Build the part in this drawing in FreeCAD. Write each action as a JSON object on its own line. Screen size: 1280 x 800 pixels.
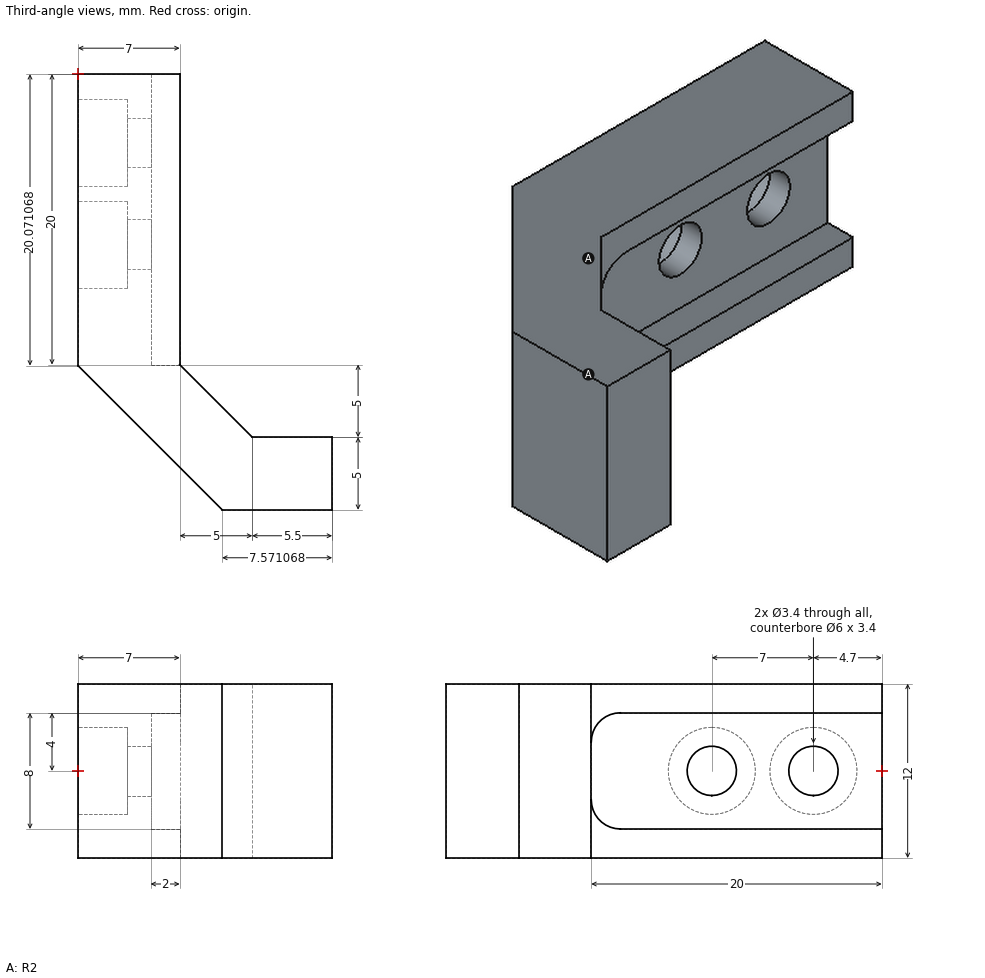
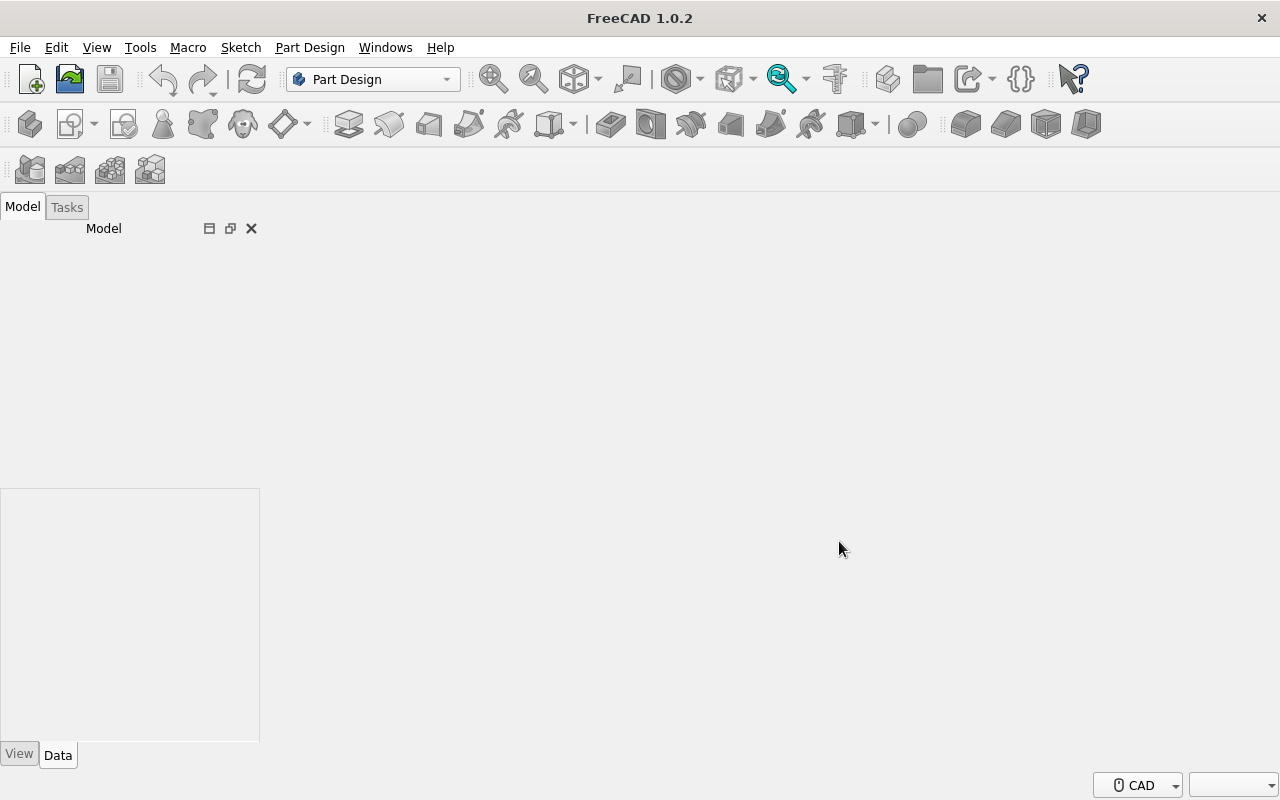
{"action": "left_click", "coordinate": [30, 80]}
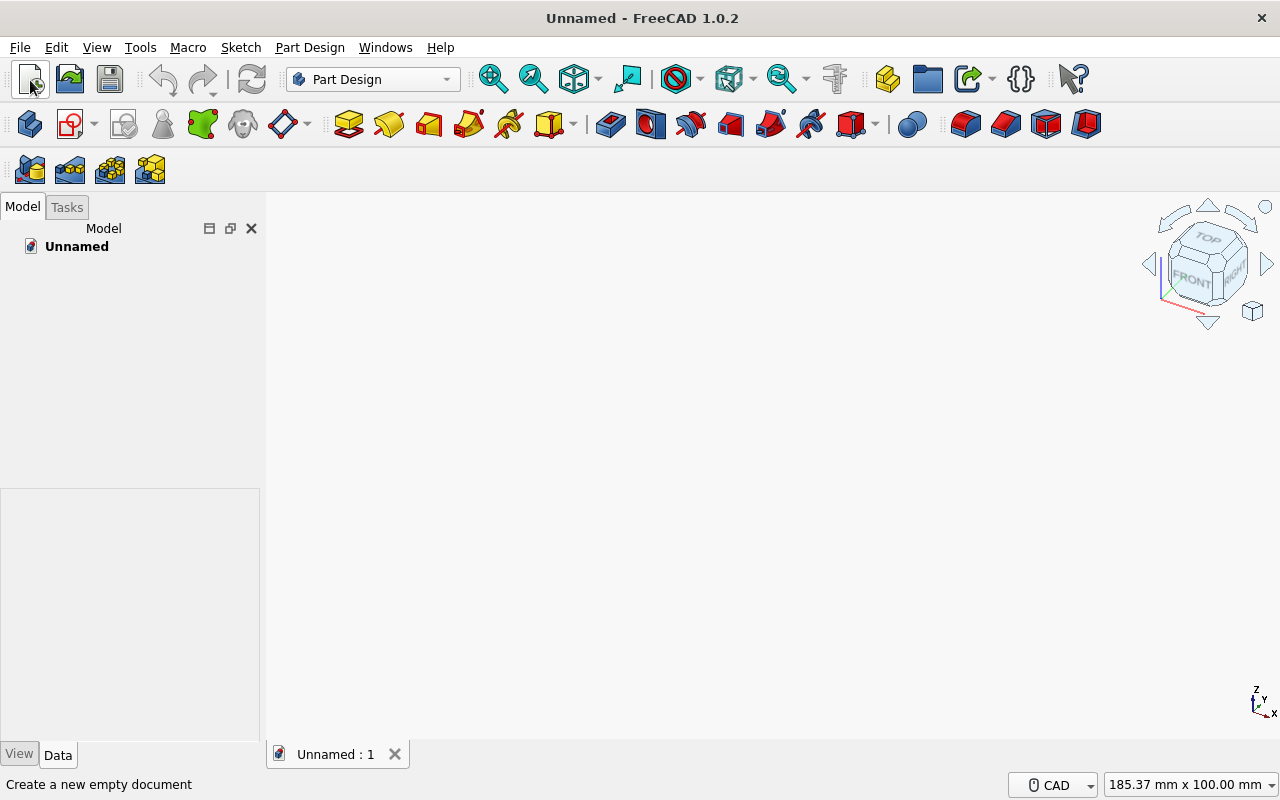
{"action": "left_click", "coordinate": [70, 124]}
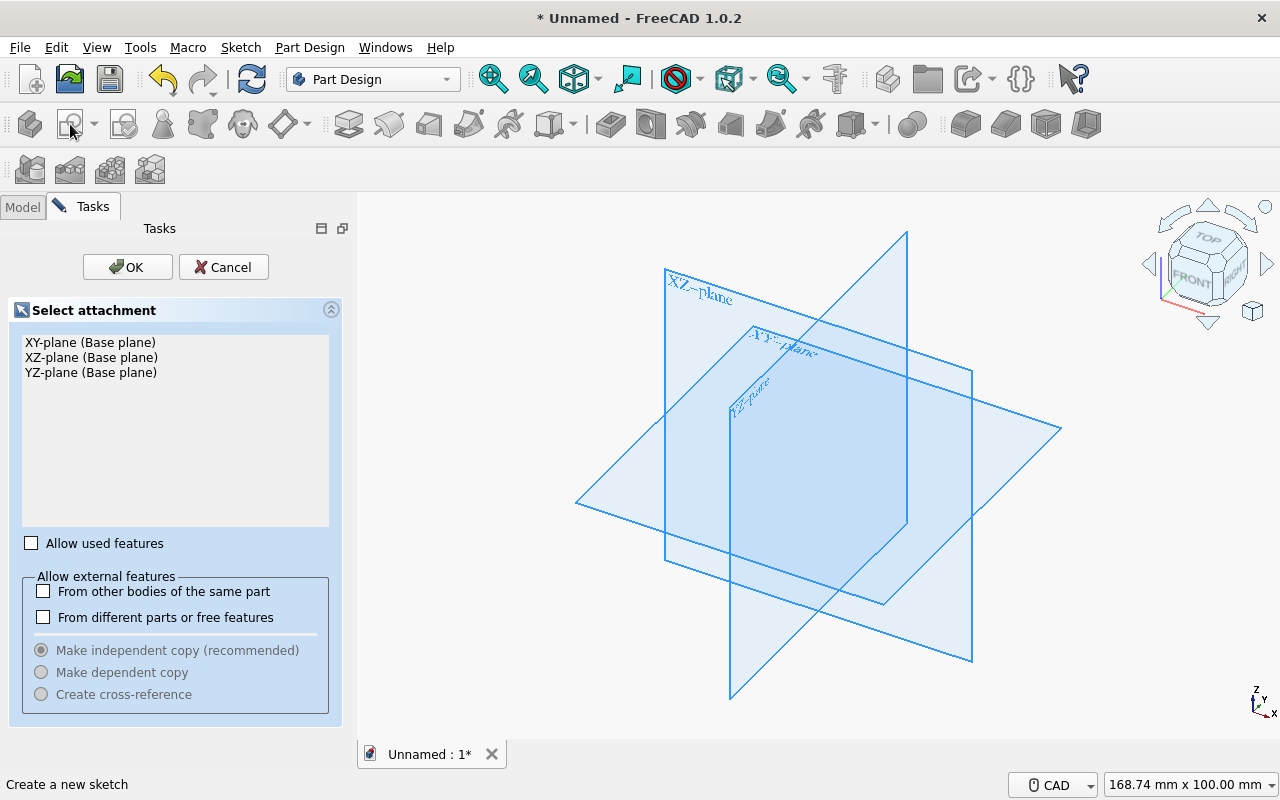
{"action": "left_click", "coordinate": [82, 342]}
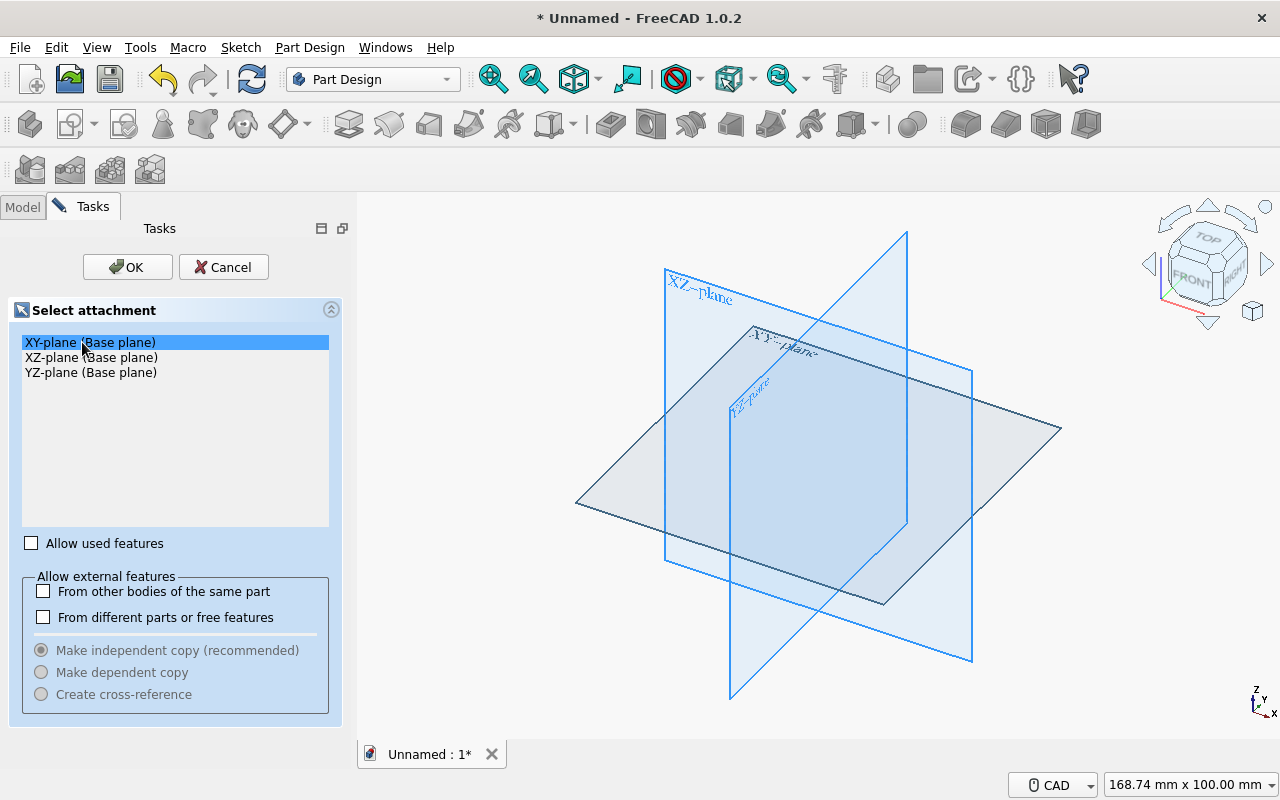
{"action": "left_click", "coordinate": [128, 267]}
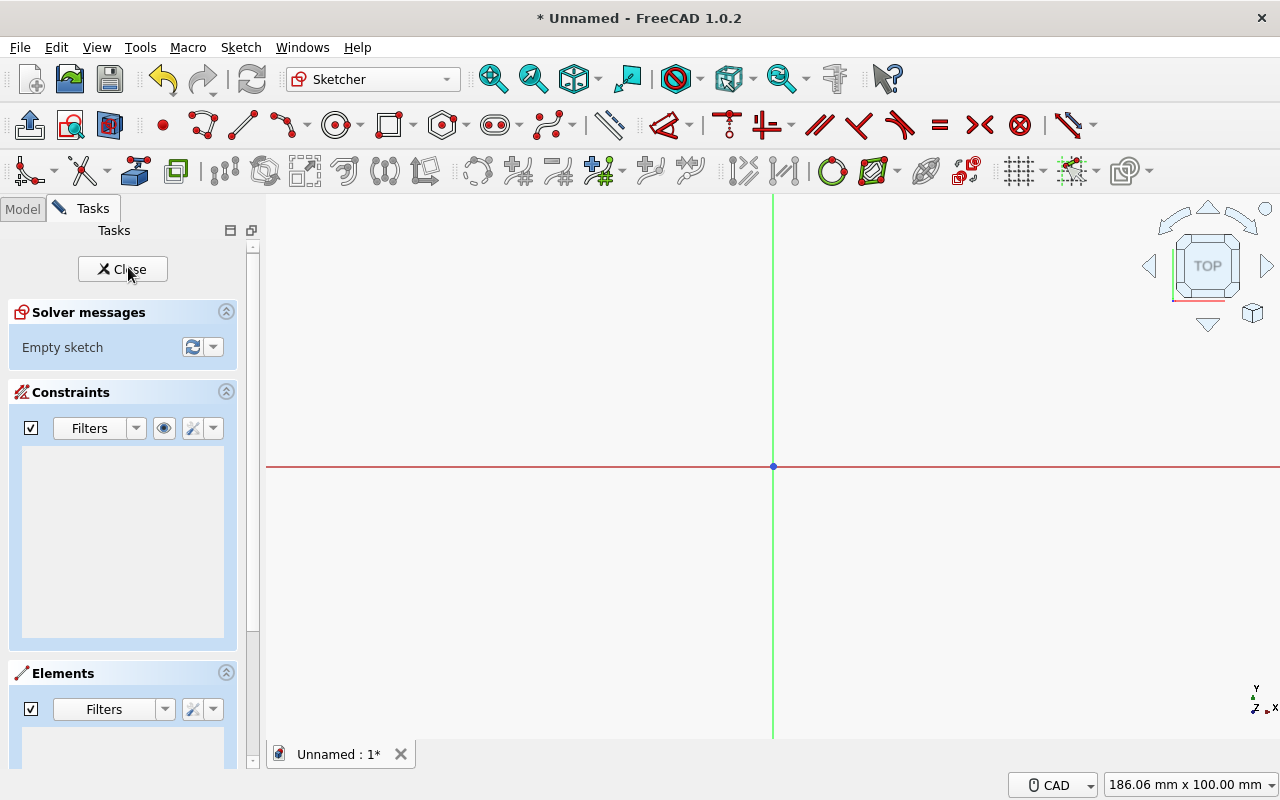
{"action": "scroll", "coordinate": [915, 615], "scroll_direction": "up", "scroll_amount": 4}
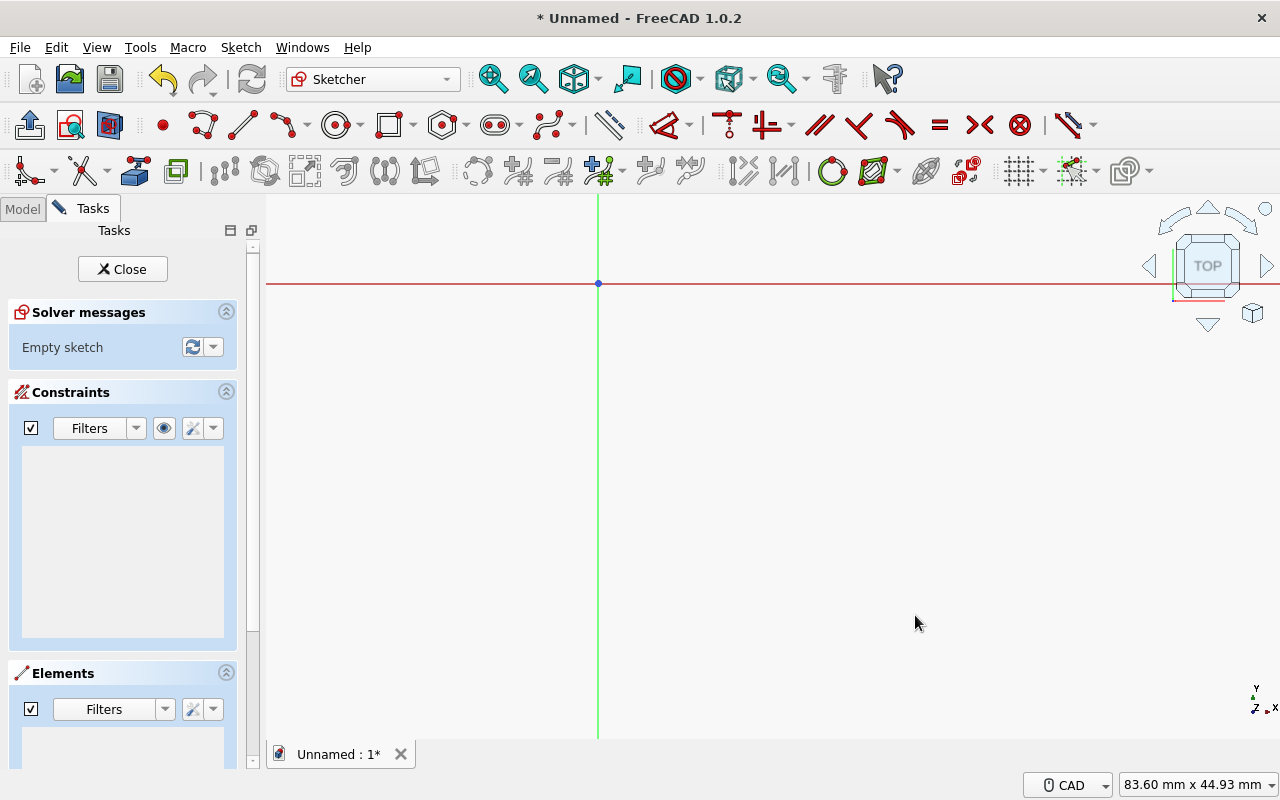
{"action": "left_click", "coordinate": [204, 126]}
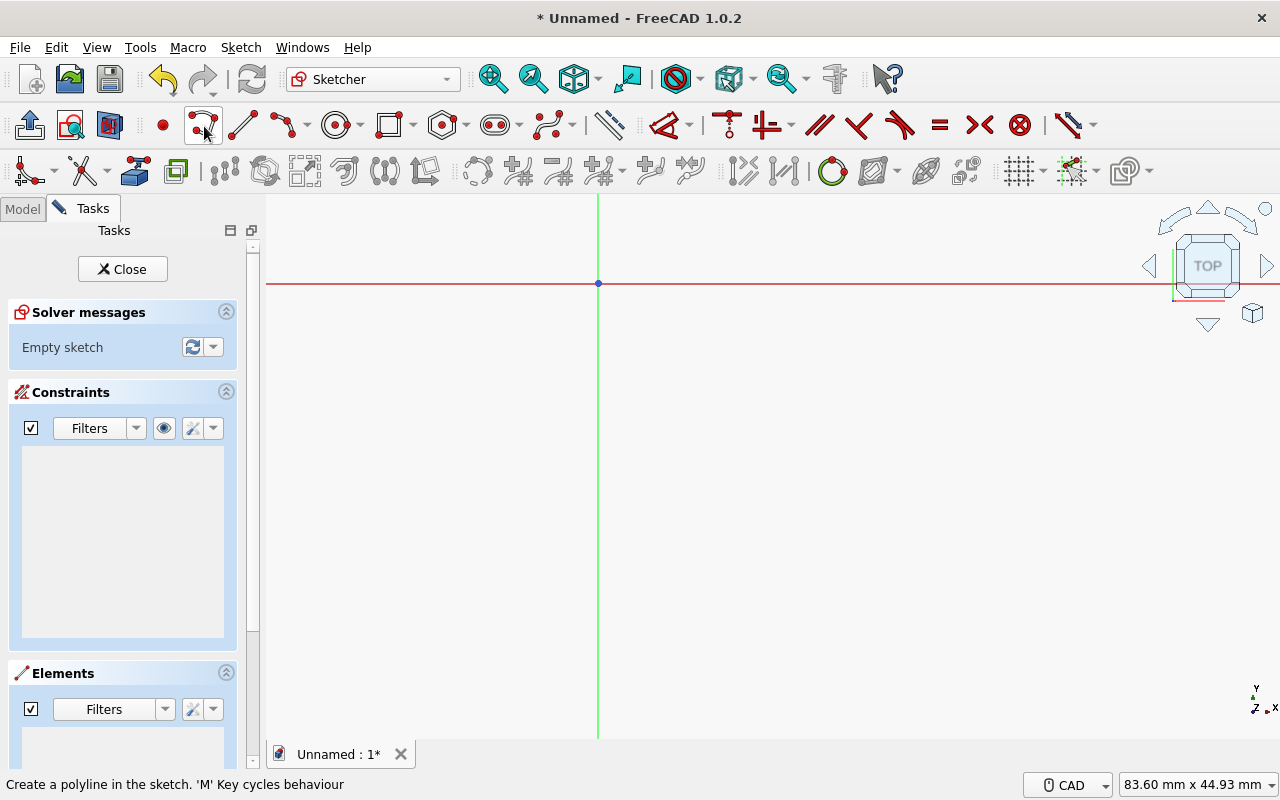
{"action": "left_click", "coordinate": [598, 284]}
{"action": "left_click", "coordinate": [607, 527]}
{"action": "left_click", "coordinate": [719, 647]}
{"action": "left_click", "coordinate": [810, 647]}
{"action": "left_click", "coordinate": [810, 587]}
{"action": "left_click", "coordinate": [744, 587]}
{"action": "left_click", "coordinate": [683, 526]}
{"action": "left_click", "coordinate": [683, 293]}
{"action": "left_click", "coordinate": [598, 284]}
{"action": "key", "text": "Escape"}
{"action": "key", "text": "Escape"}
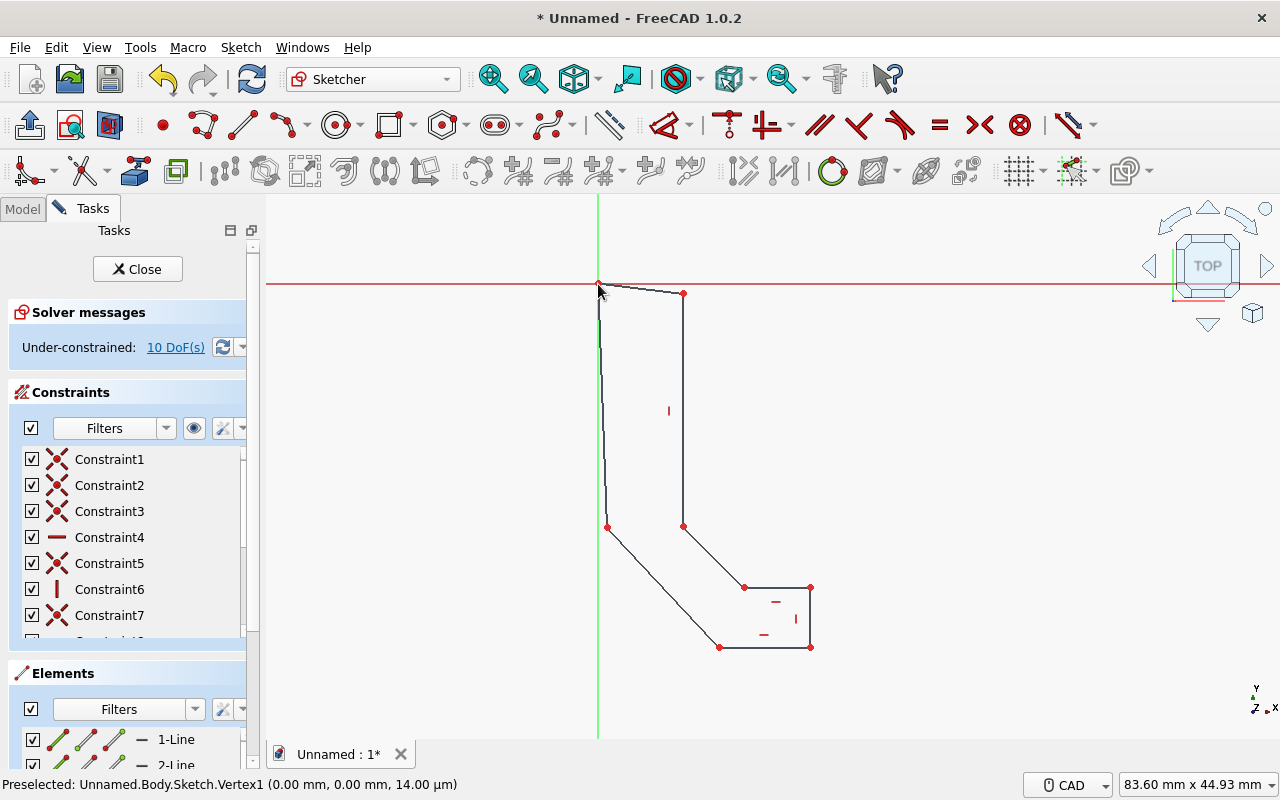
{"action": "left_click", "coordinate": [601, 357]}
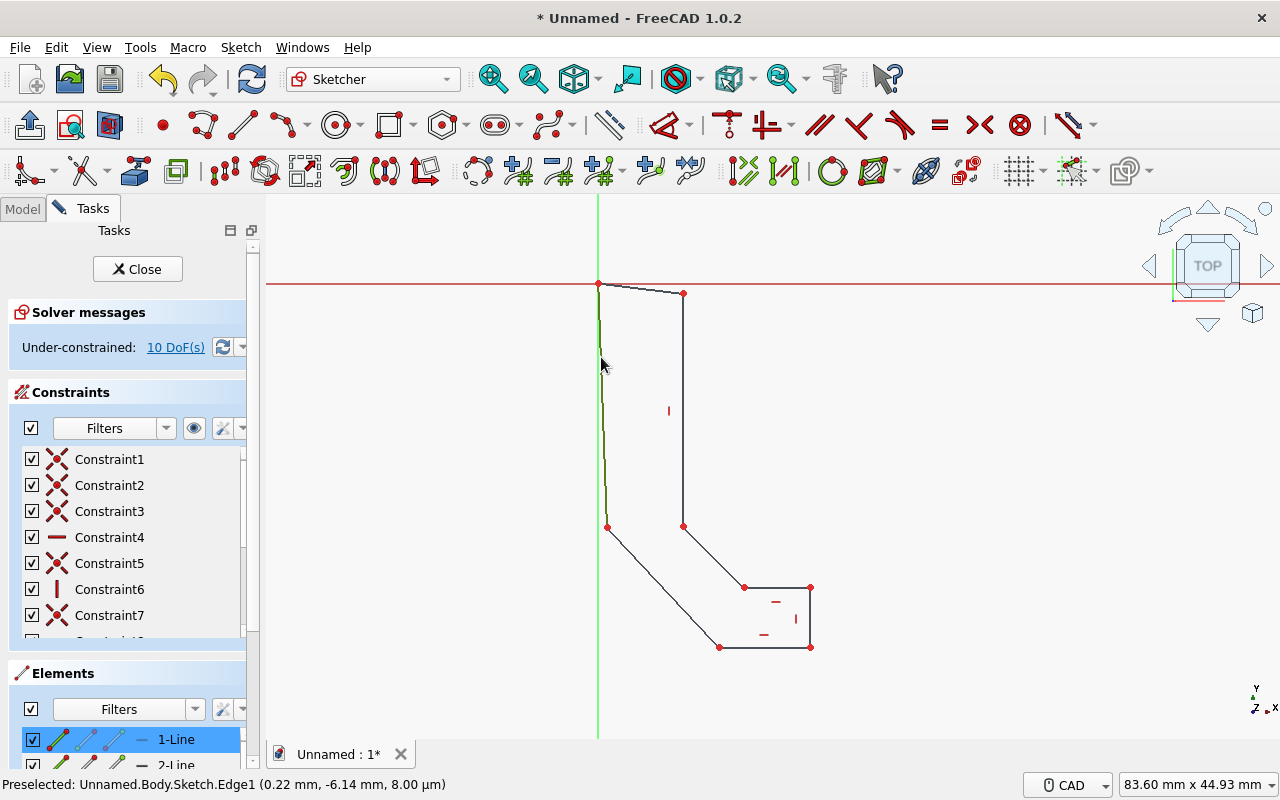
{"action": "key", "text": "v"}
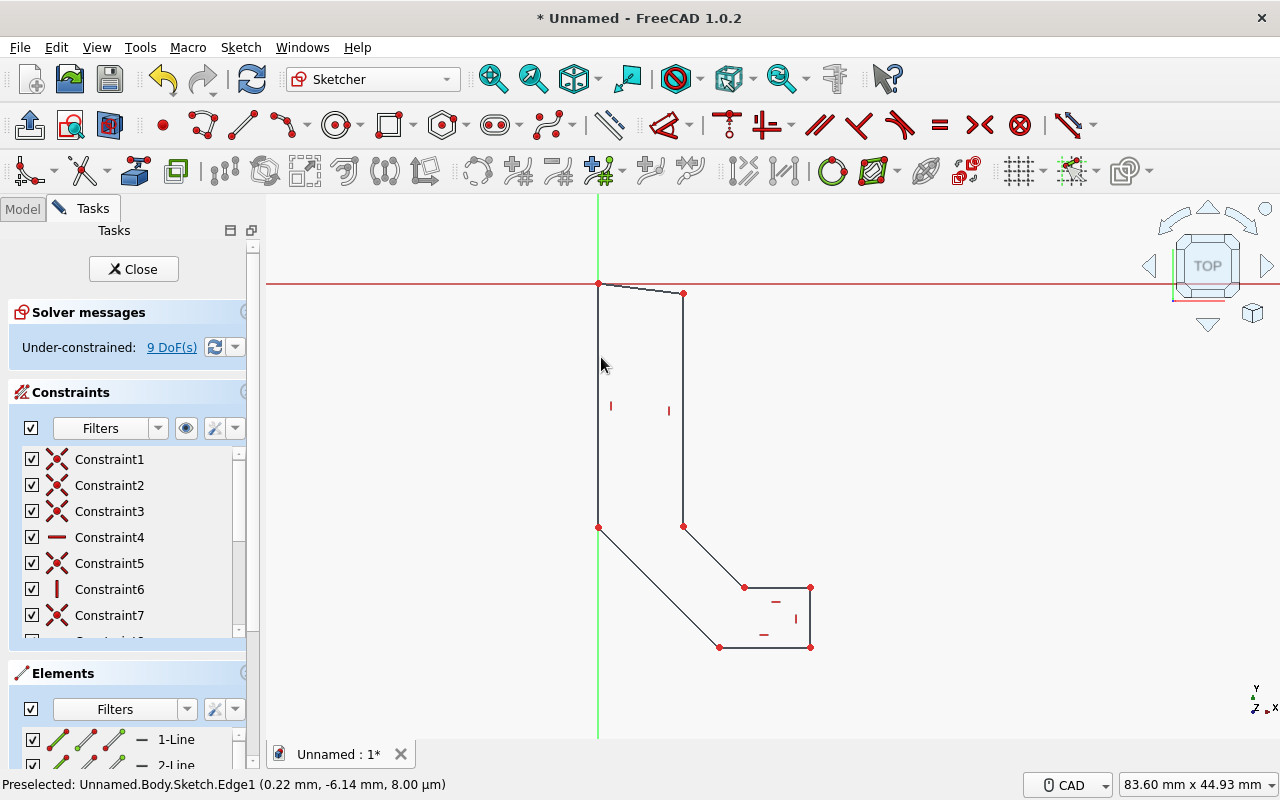
{"action": "left_click", "coordinate": [624, 287]}